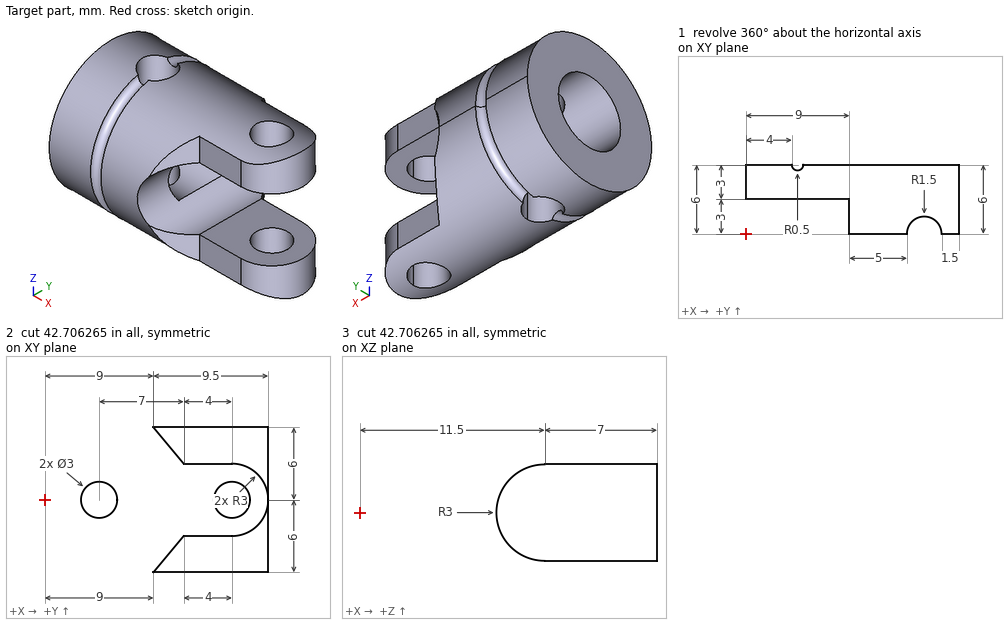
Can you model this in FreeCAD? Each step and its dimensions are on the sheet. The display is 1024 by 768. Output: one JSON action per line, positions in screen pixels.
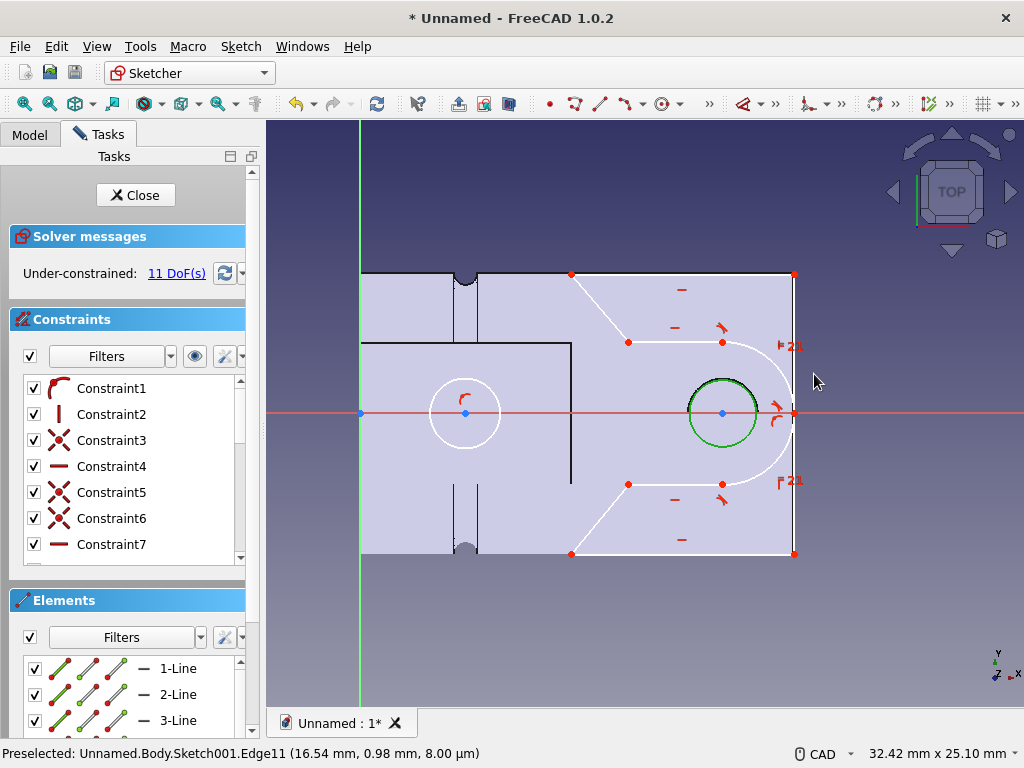
{"action": "left_click", "coordinate": [490, 389]}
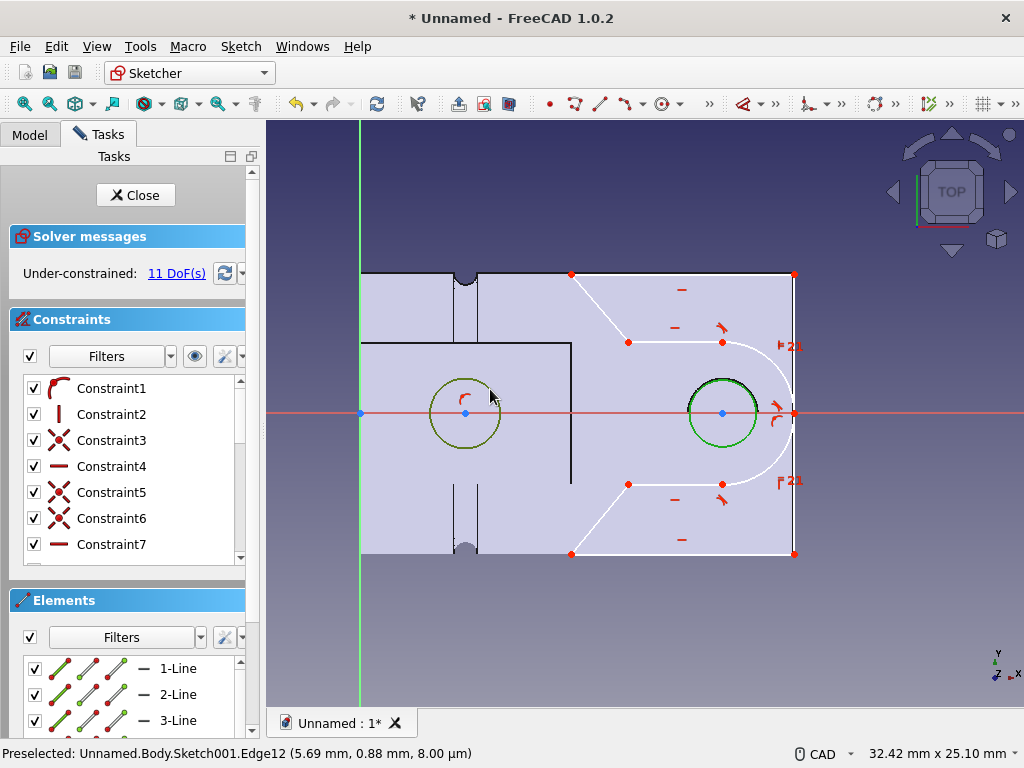
{"action": "key", "text": "e"}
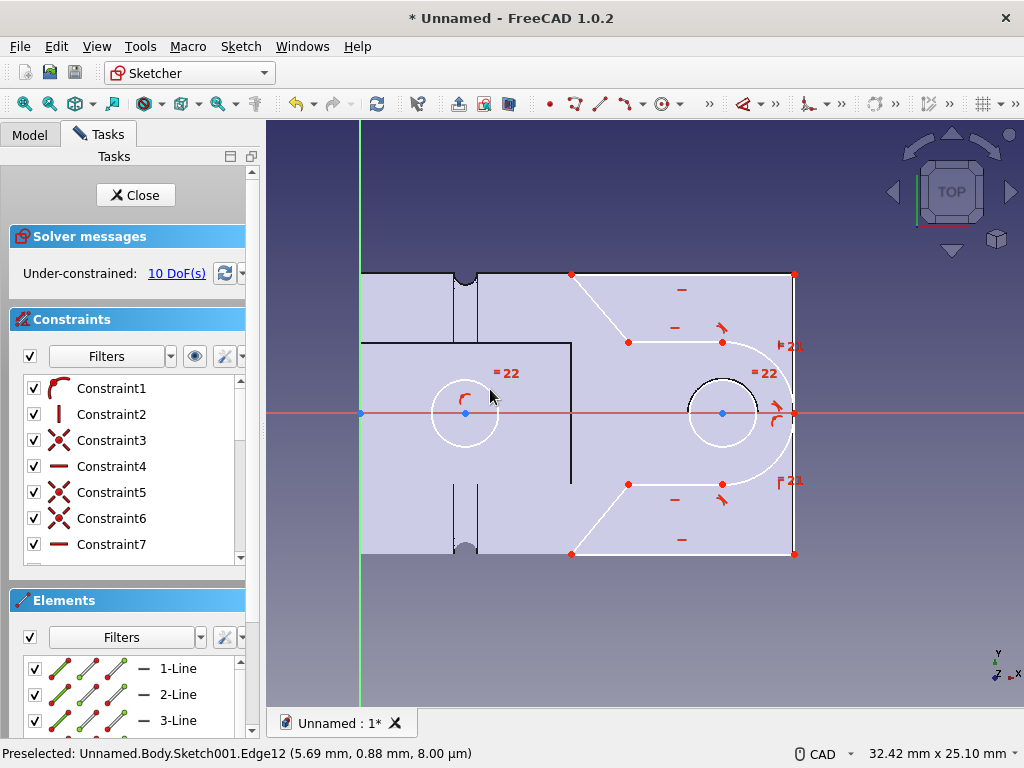
{"action": "left_click", "coordinate": [742, 104]}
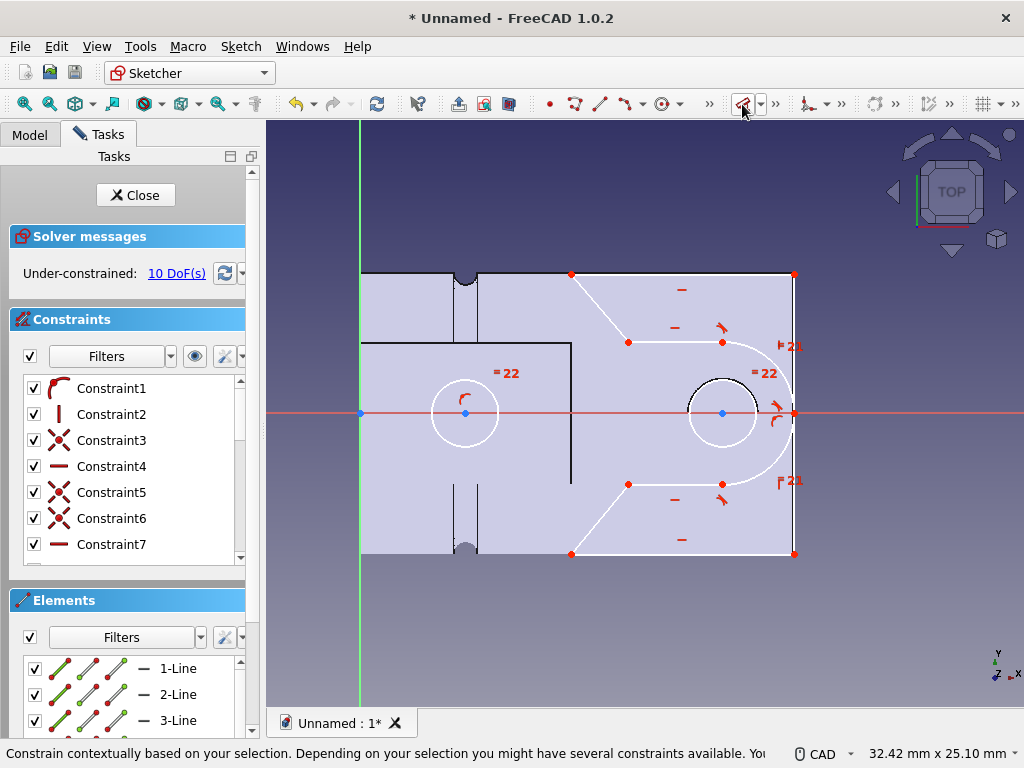
{"action": "left_click", "coordinate": [755, 350]}
{"action": "left_click", "coordinate": [769, 321]}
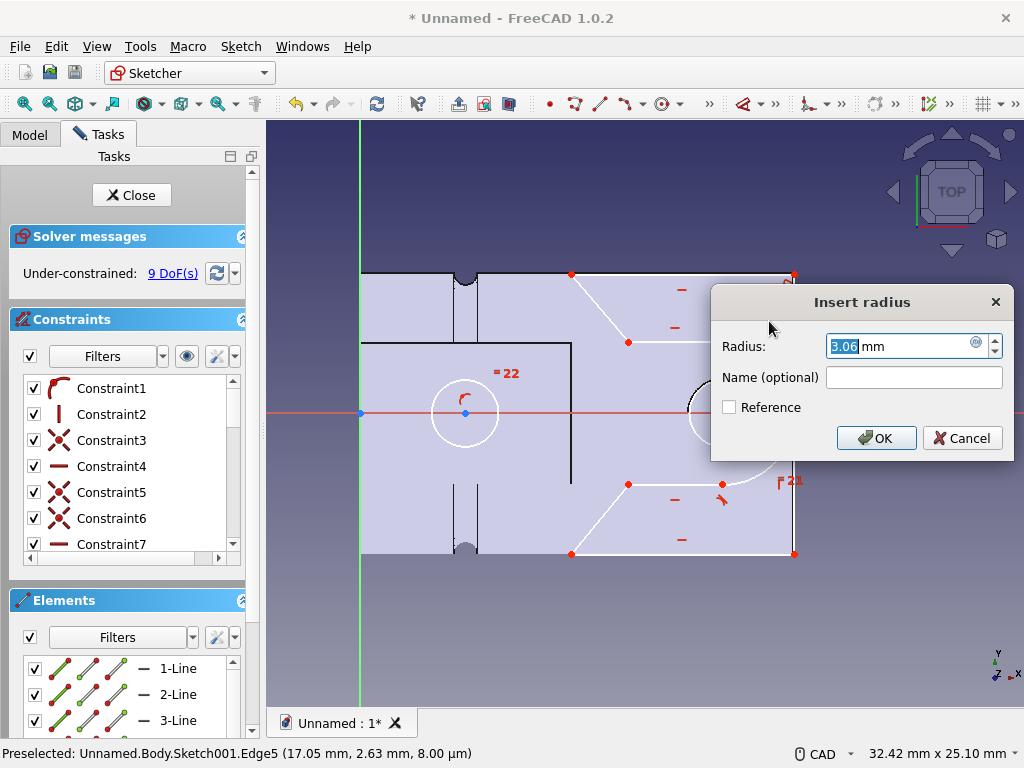
{"action": "type", "text": "3"}
{"action": "key", "text": "Return"}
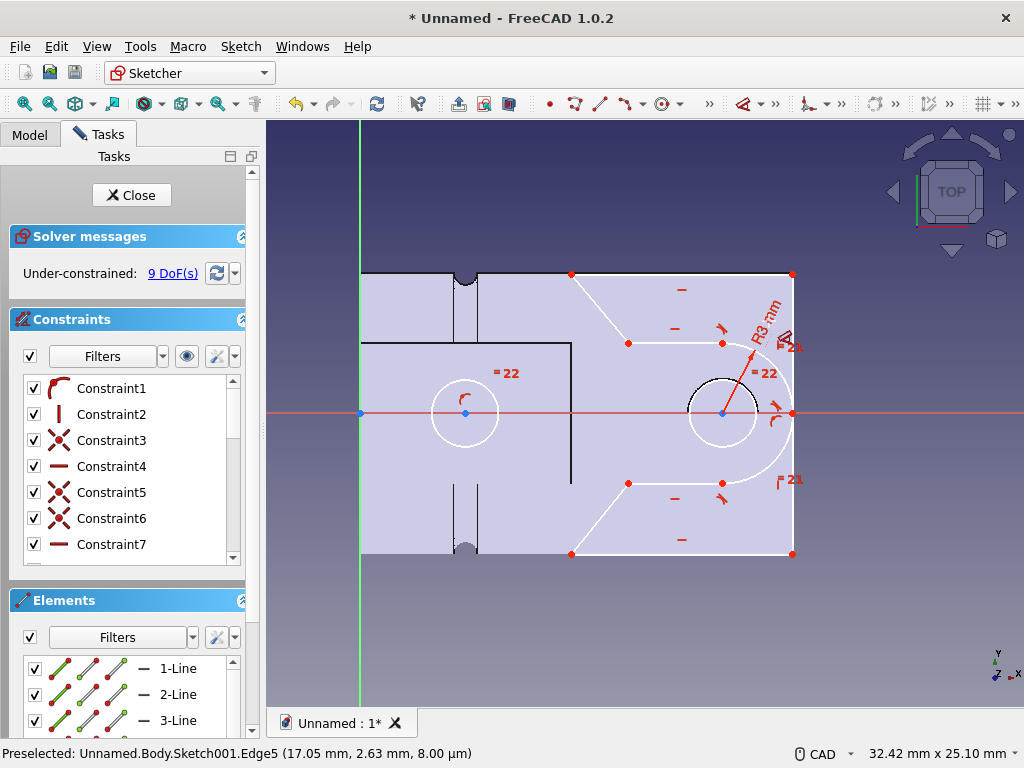
{"action": "left_click", "coordinate": [746, 390]}
{"action": "left_click", "coordinate": [677, 368]}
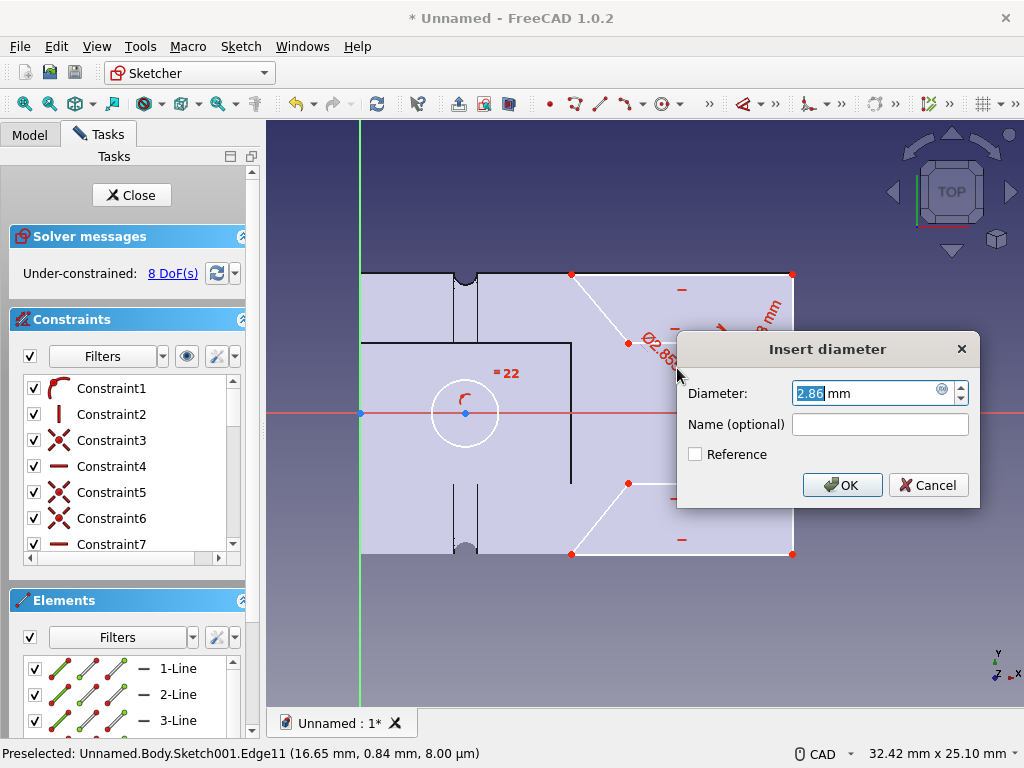
{"action": "type", "text": "3"}
{"action": "key", "text": "Return"}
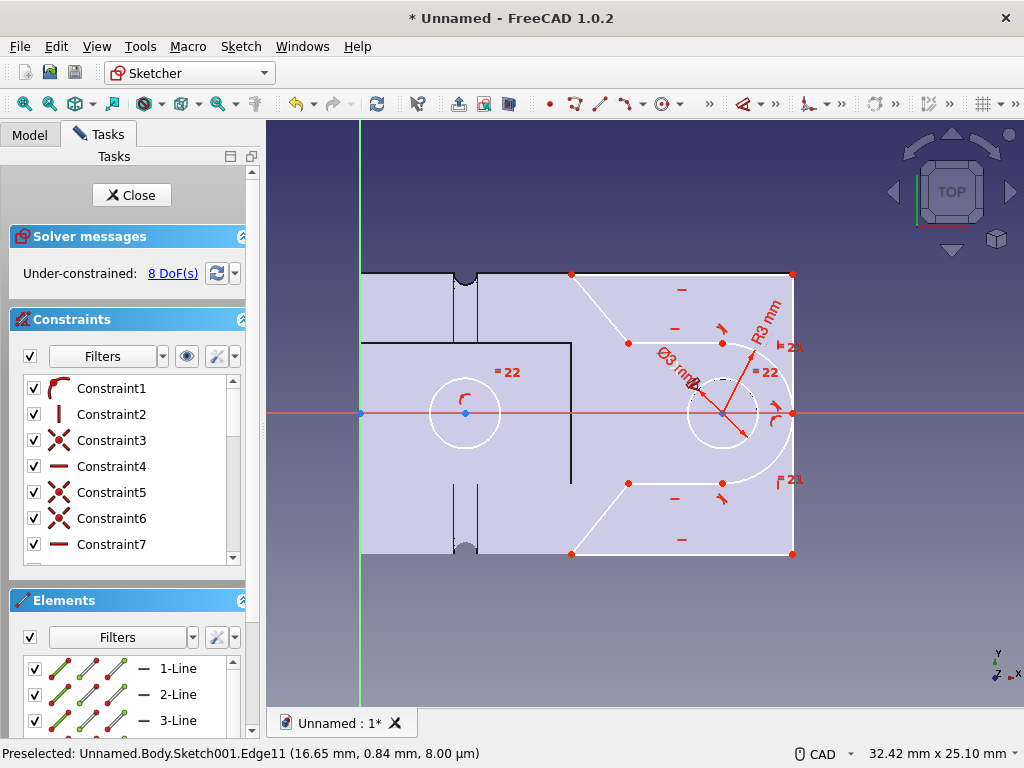
{"action": "left_click", "coordinate": [793, 372]}
{"action": "left_click", "coordinate": [827, 344]}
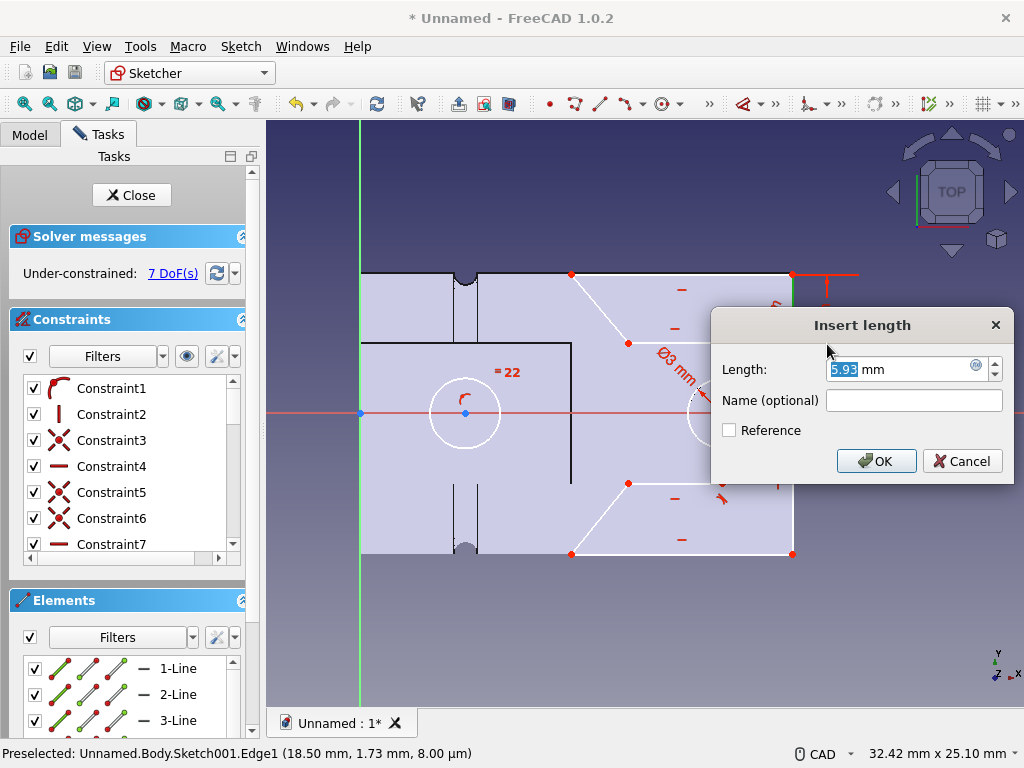
{"action": "type", "text": "6"}
{"action": "key", "text": "Return"}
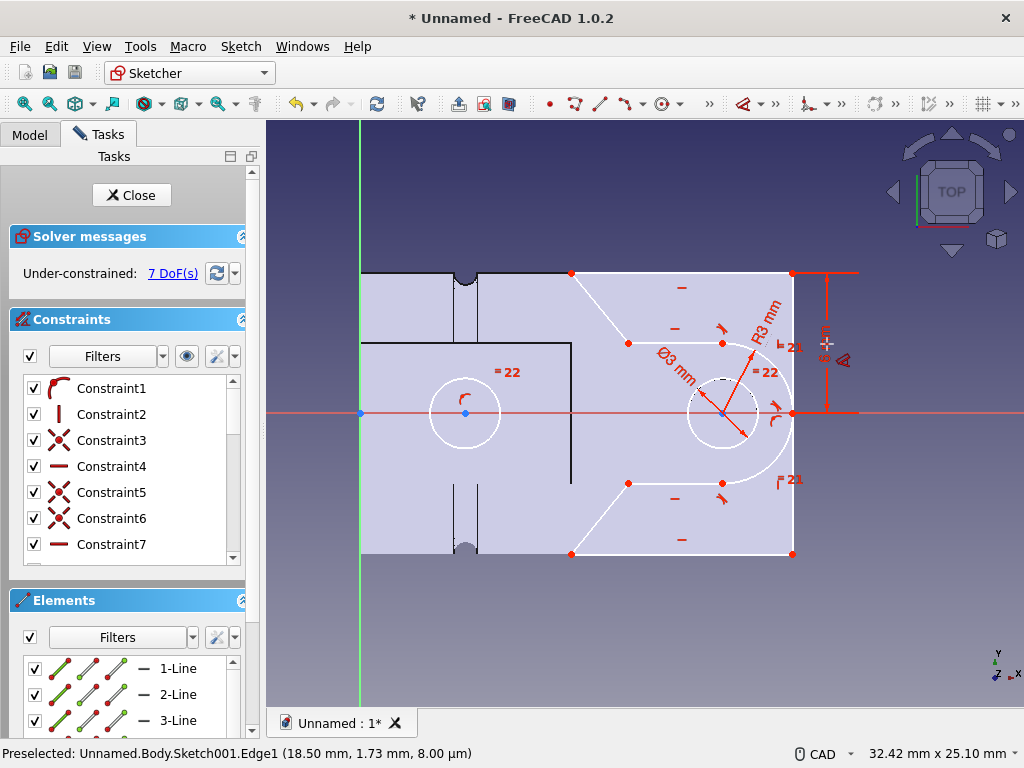
{"action": "left_click", "coordinate": [657, 343]}
{"action": "left_click", "coordinate": [676, 309]}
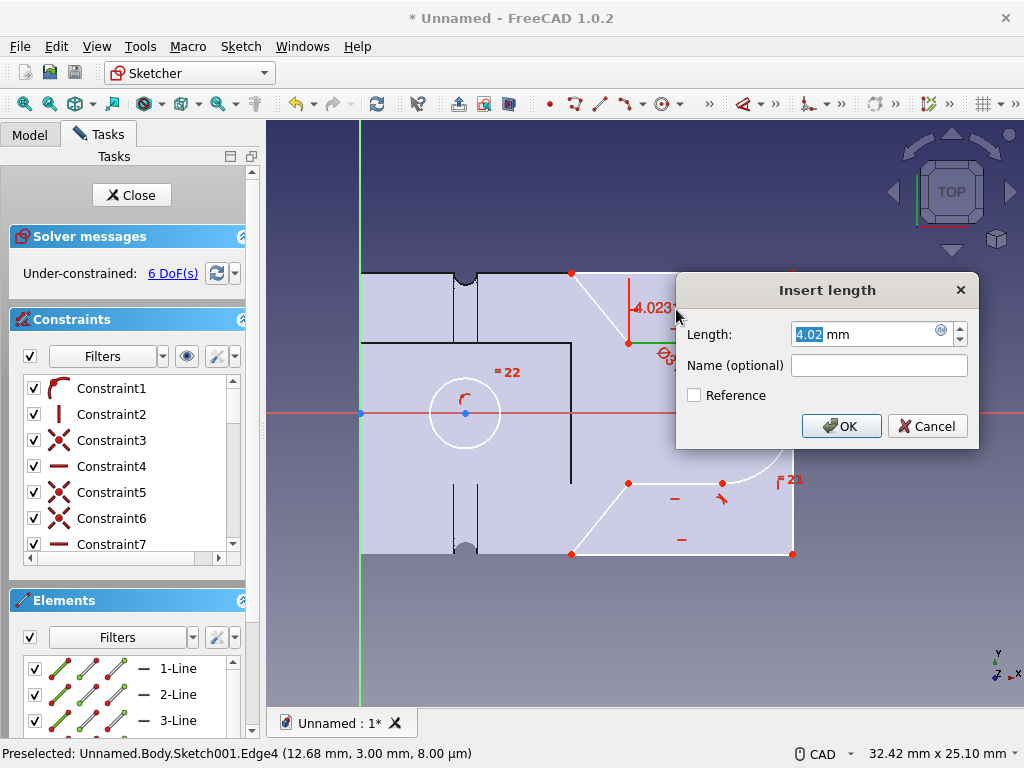
{"action": "type", "text": "4"}
{"action": "key", "text": "Return"}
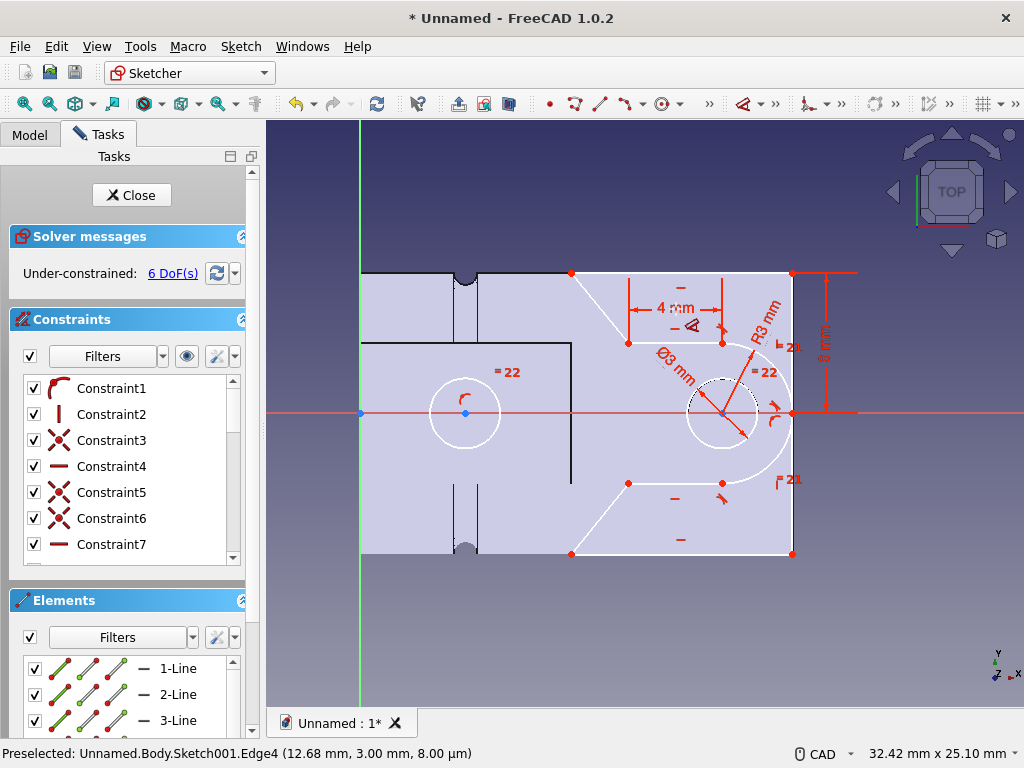
{"action": "left_click", "coordinate": [694, 484]}
{"action": "left_click", "coordinate": [676, 518]}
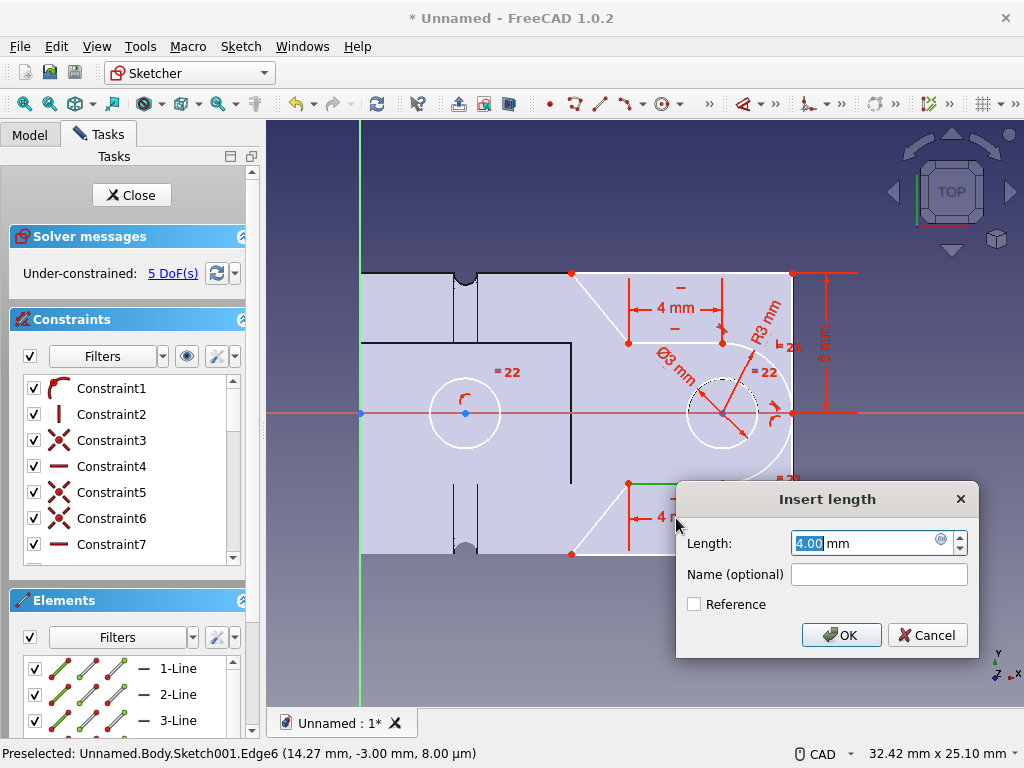
{"action": "type", "text": "4"}
{"action": "key", "text": "Return"}